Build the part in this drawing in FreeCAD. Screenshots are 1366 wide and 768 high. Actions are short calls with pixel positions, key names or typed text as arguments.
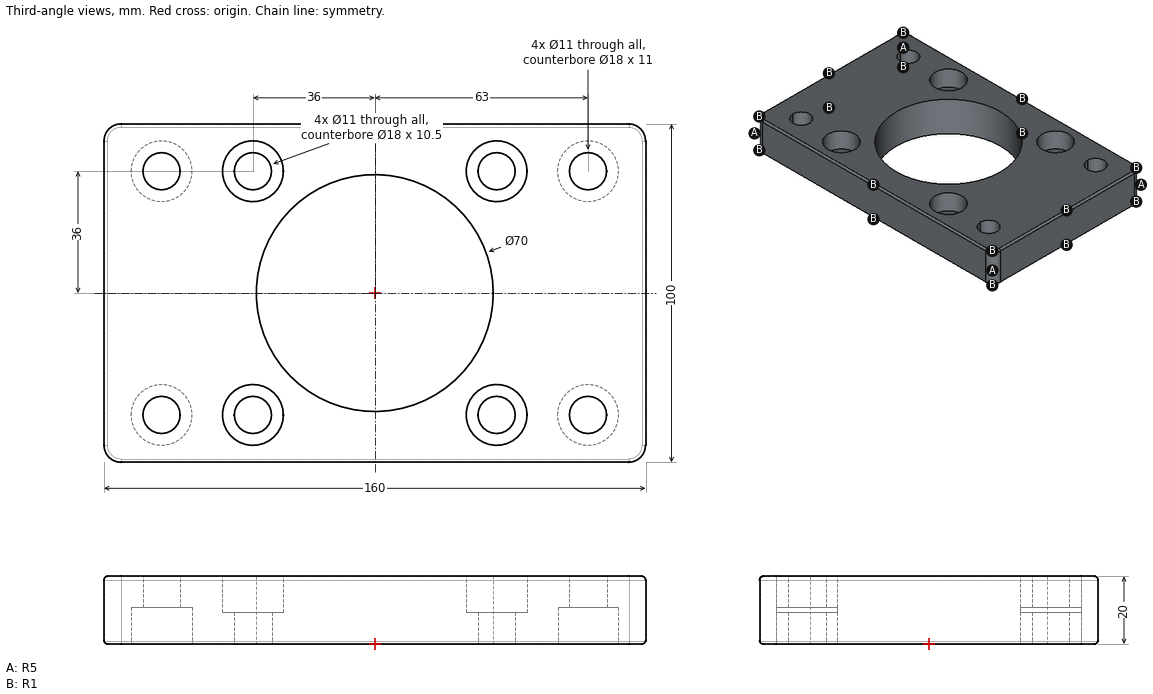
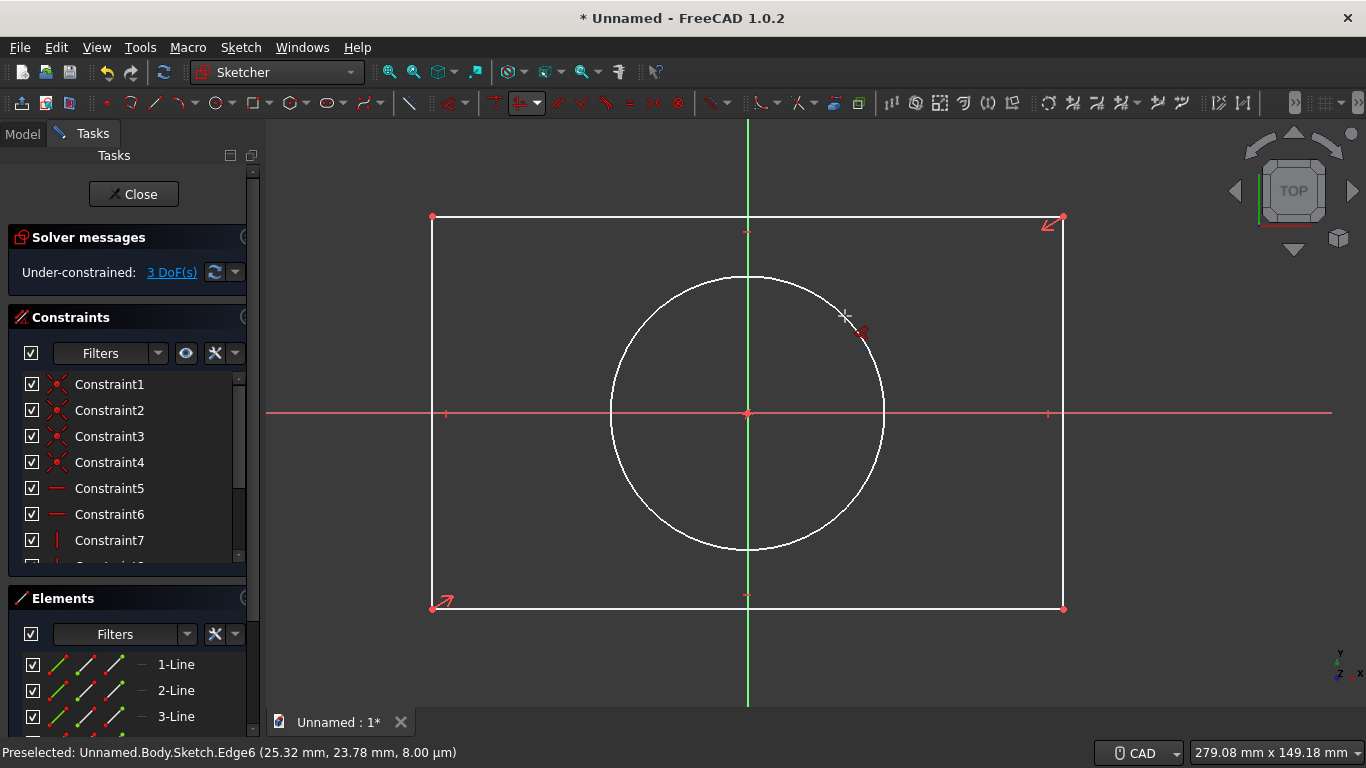
click(844, 316)
click(867, 293)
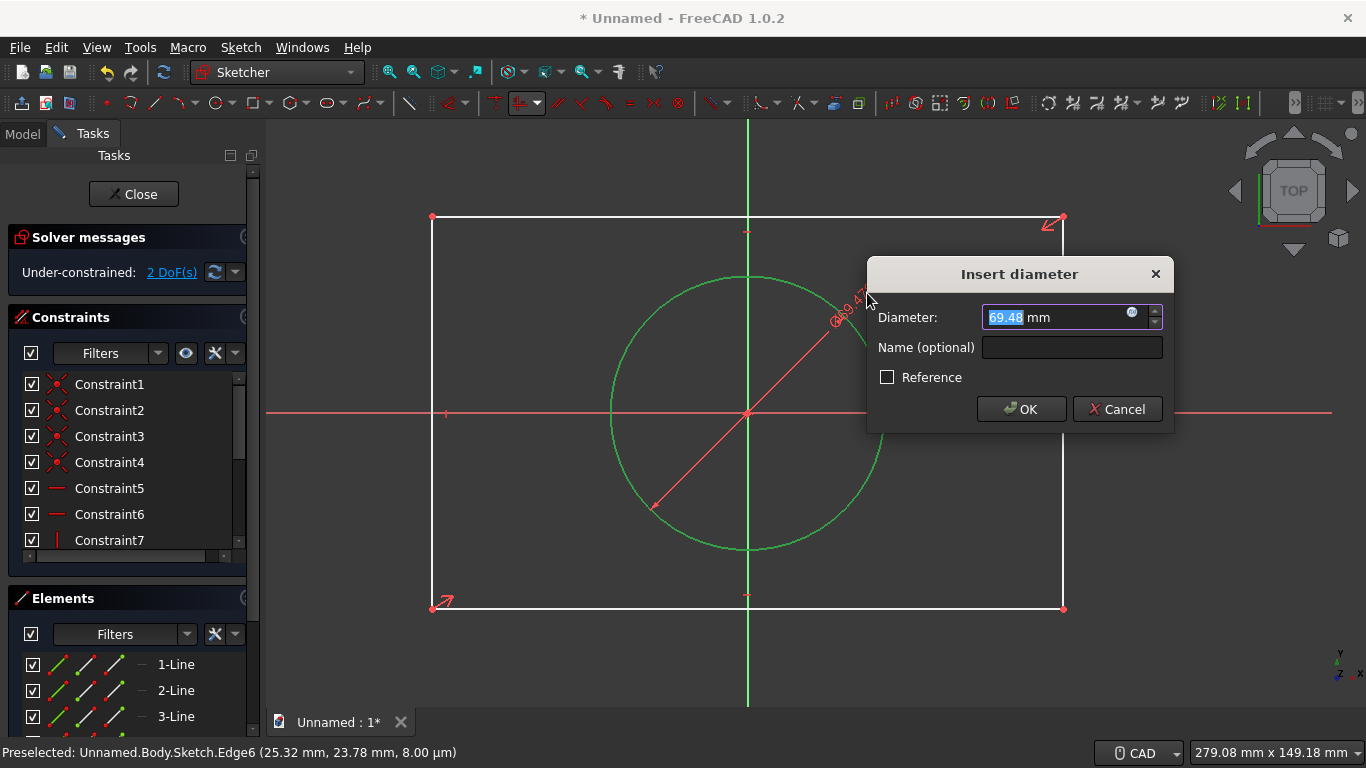
text(70)
key(Return)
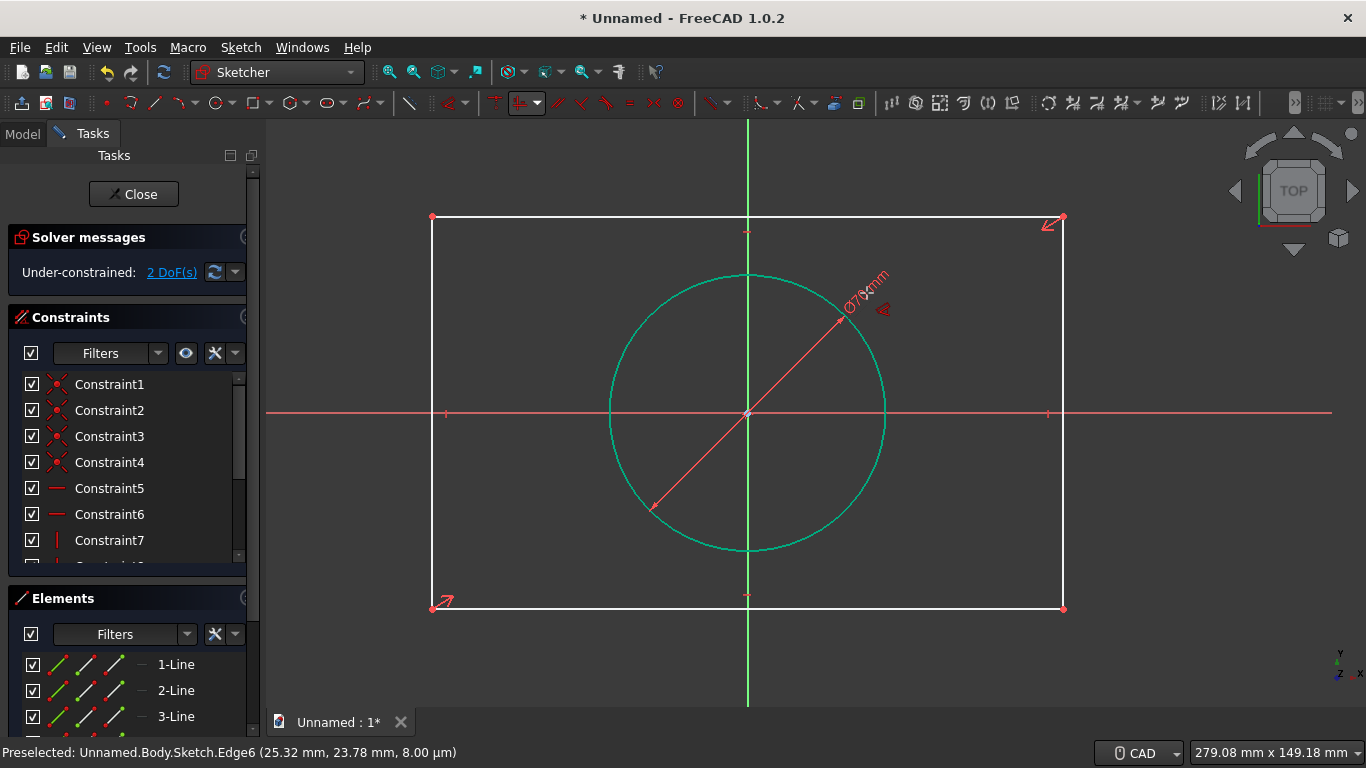
click(621, 609)
click(602, 643)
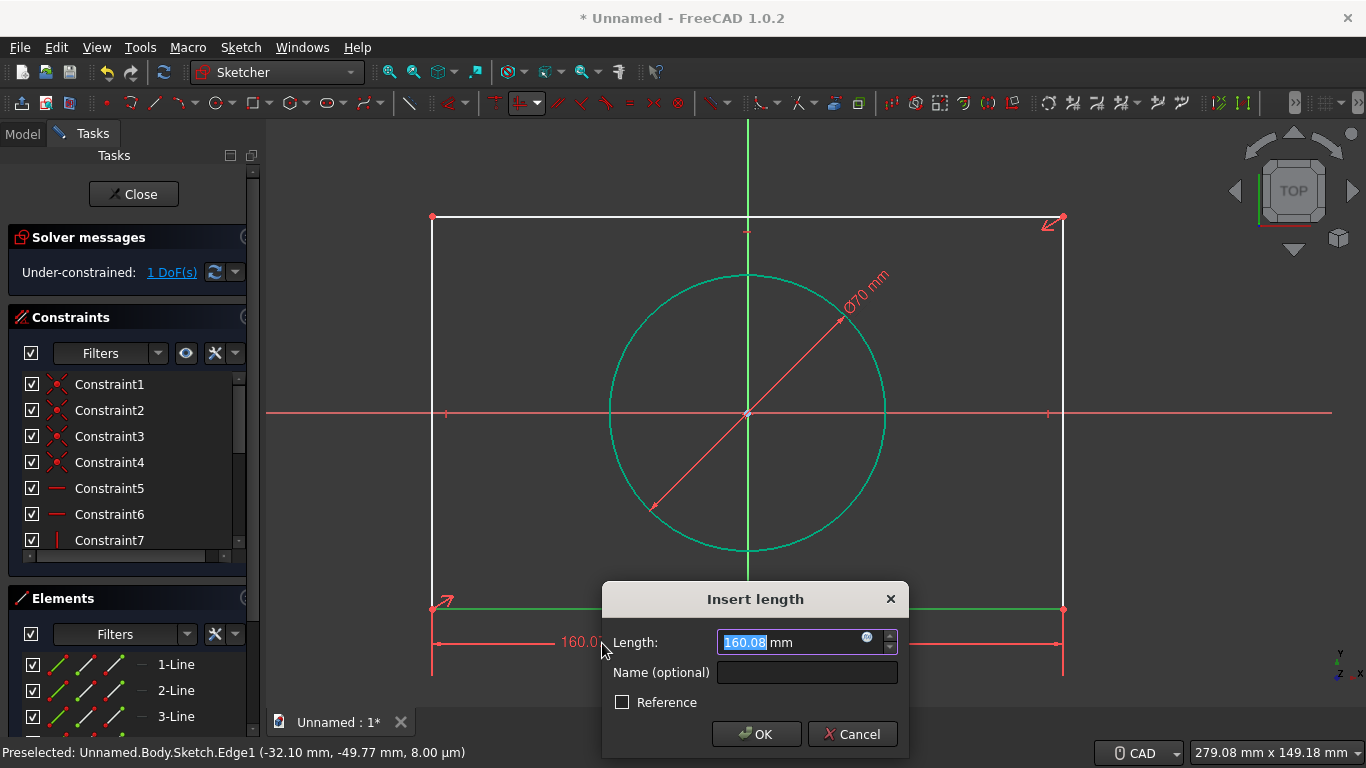
text(160)
key(Return)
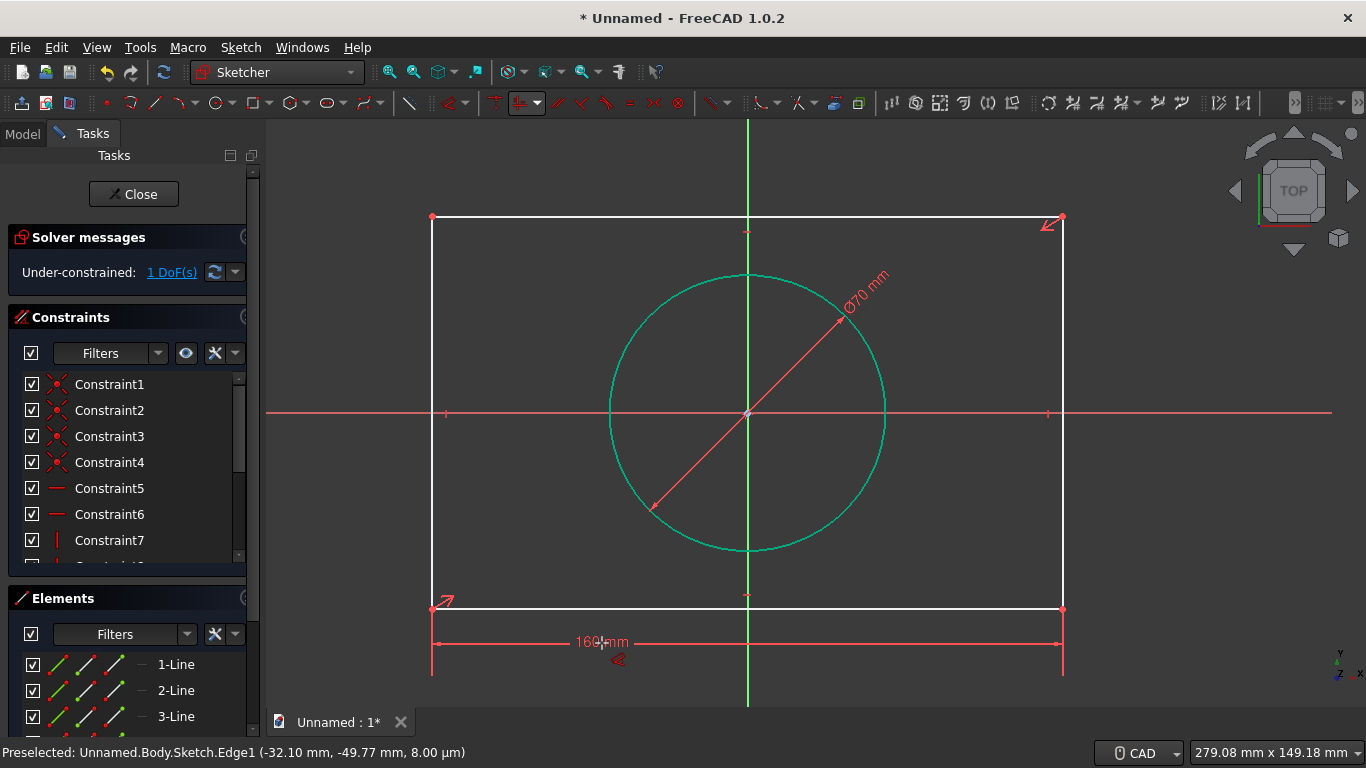
click(1063, 492)
click(1097, 323)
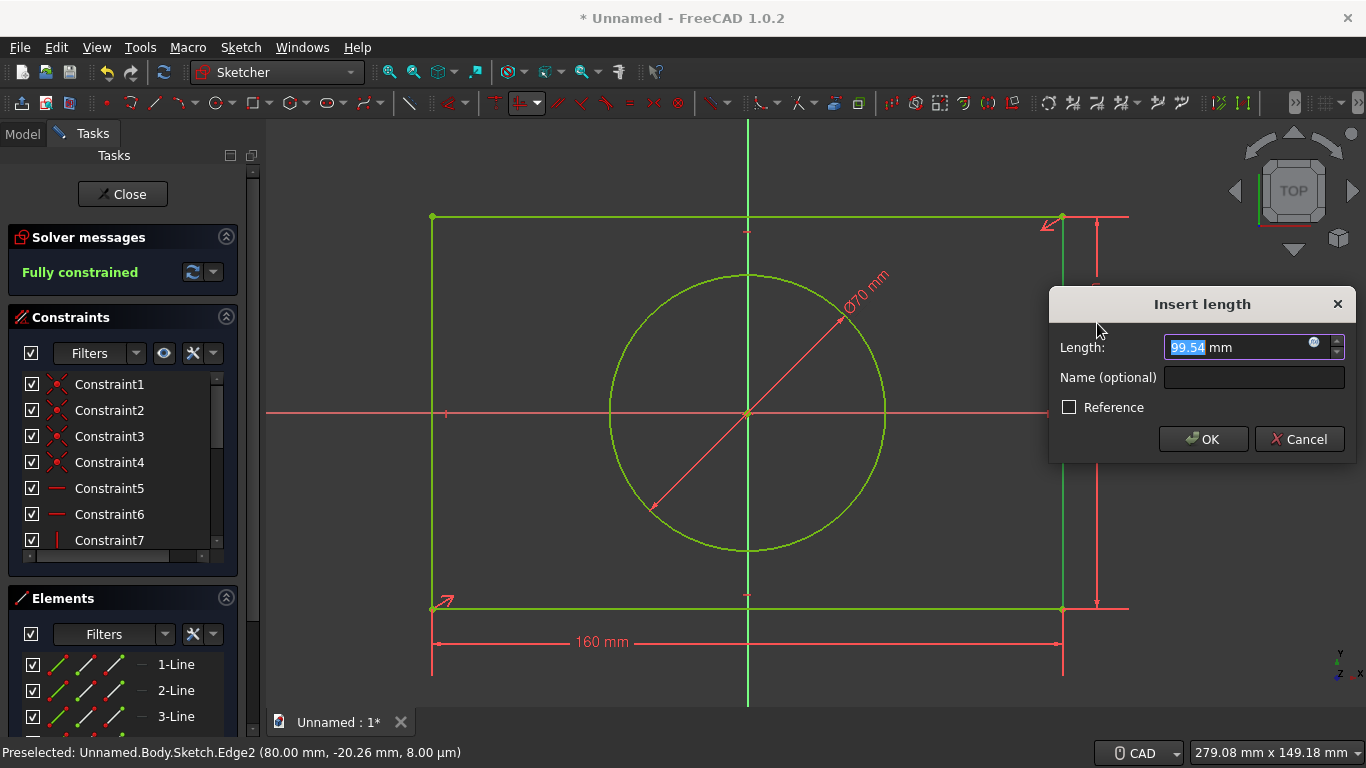
text(100)
key(Return)
key(Escape)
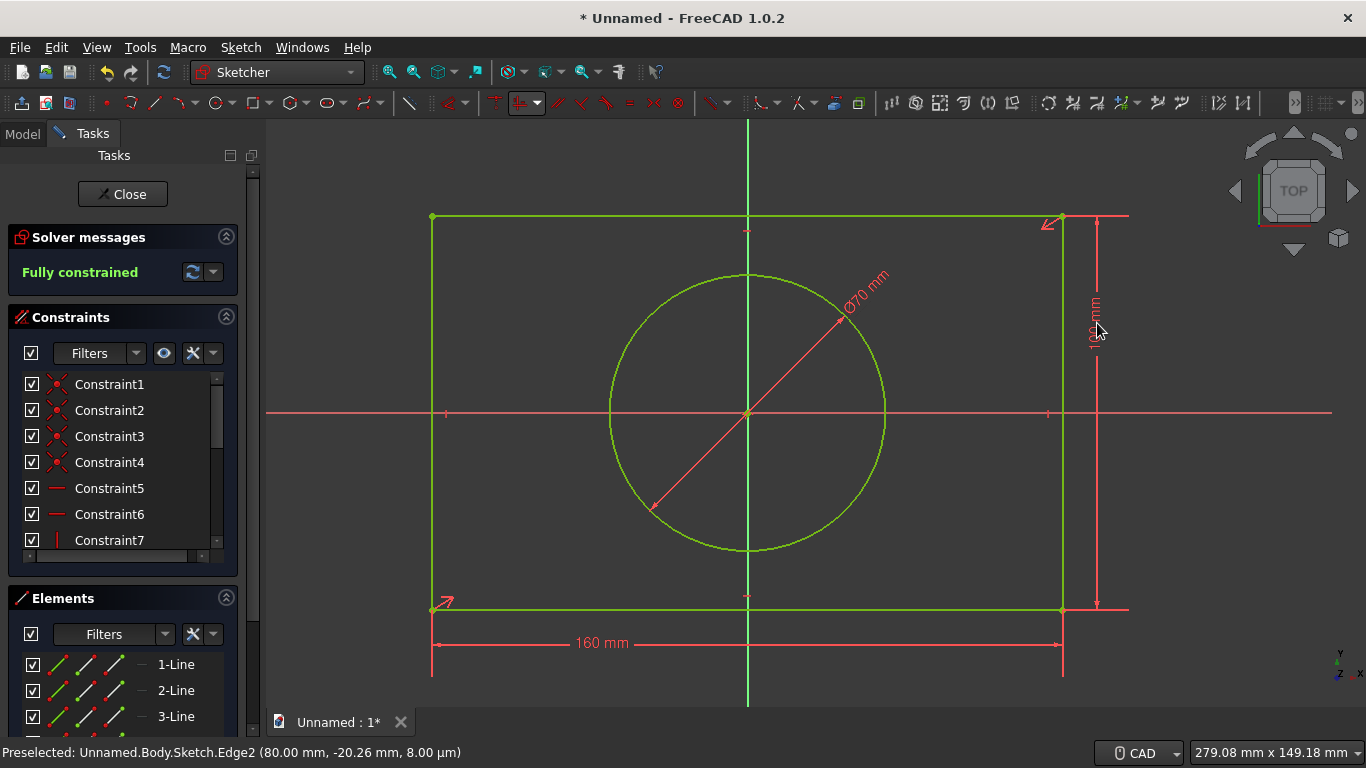
click(123, 194)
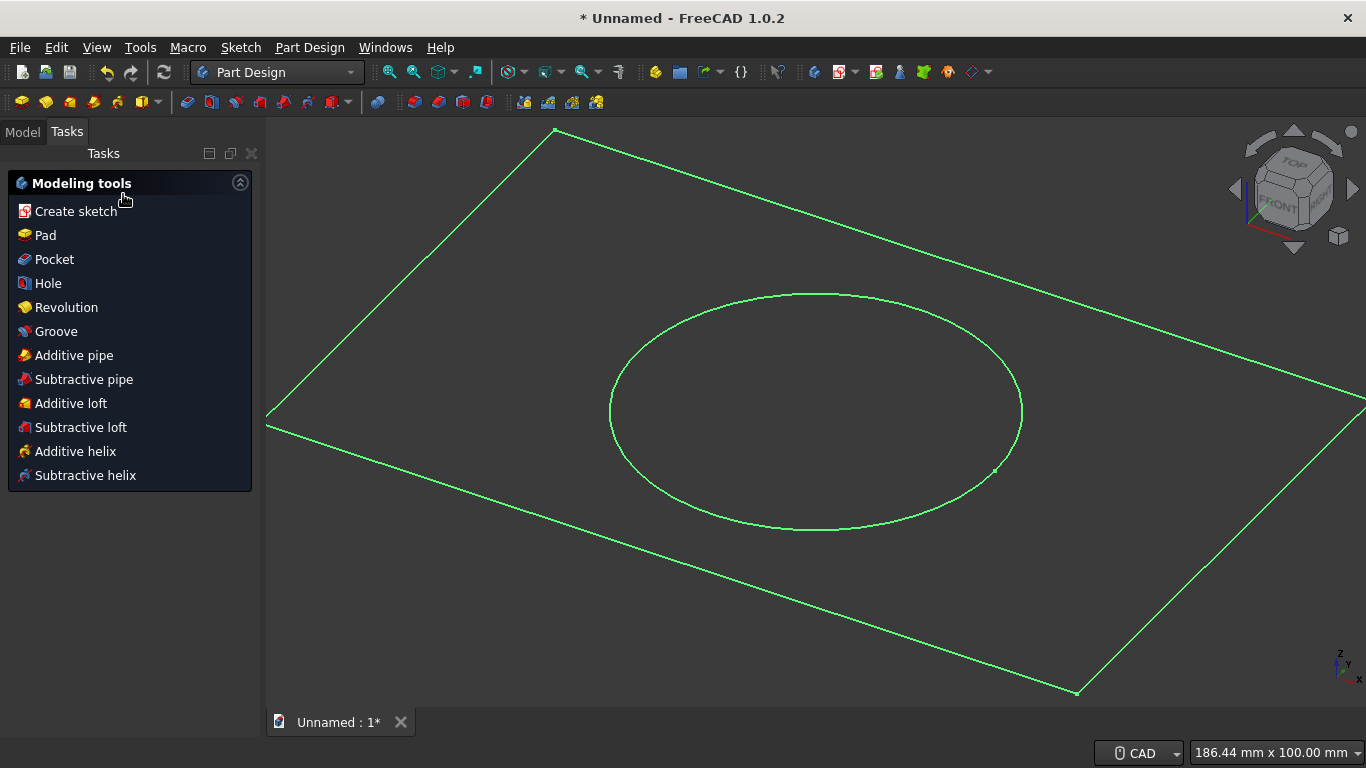
click(22, 102)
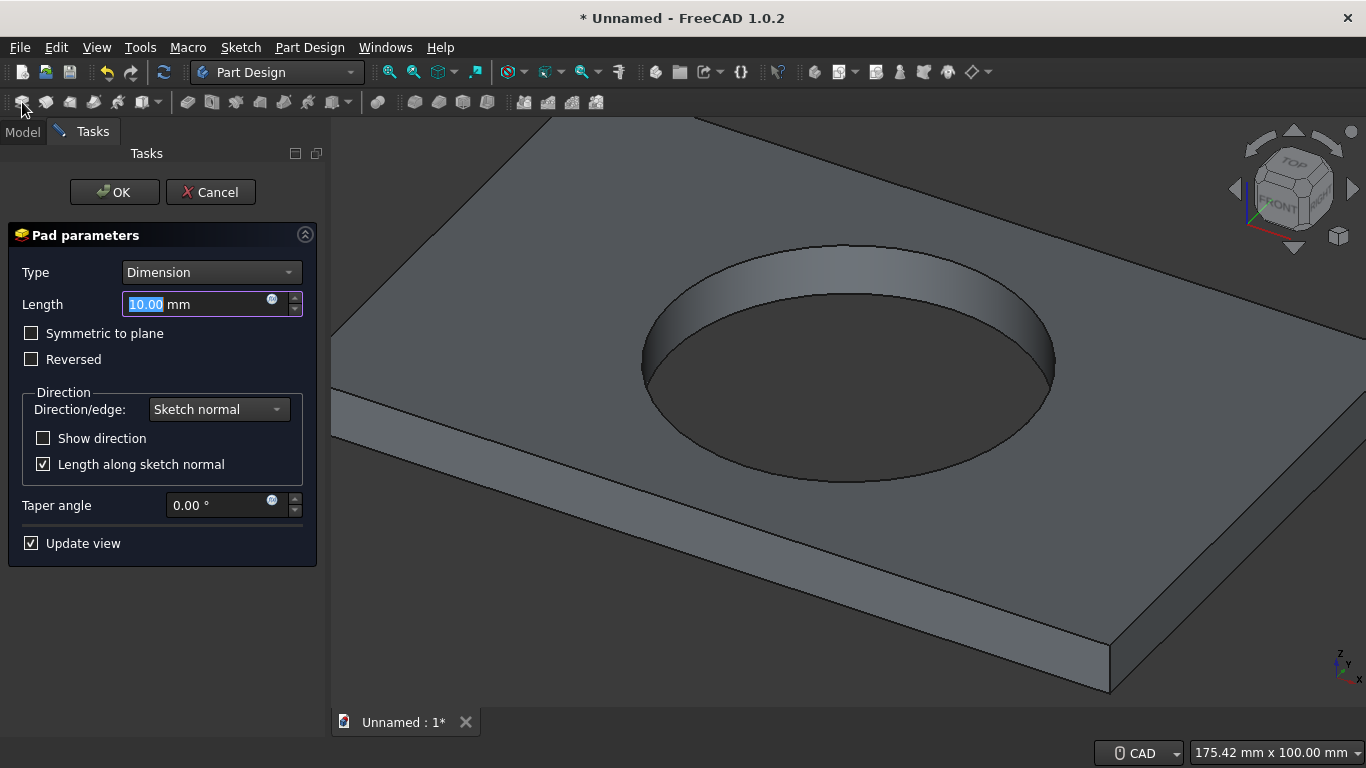
text(20)
key(Tab)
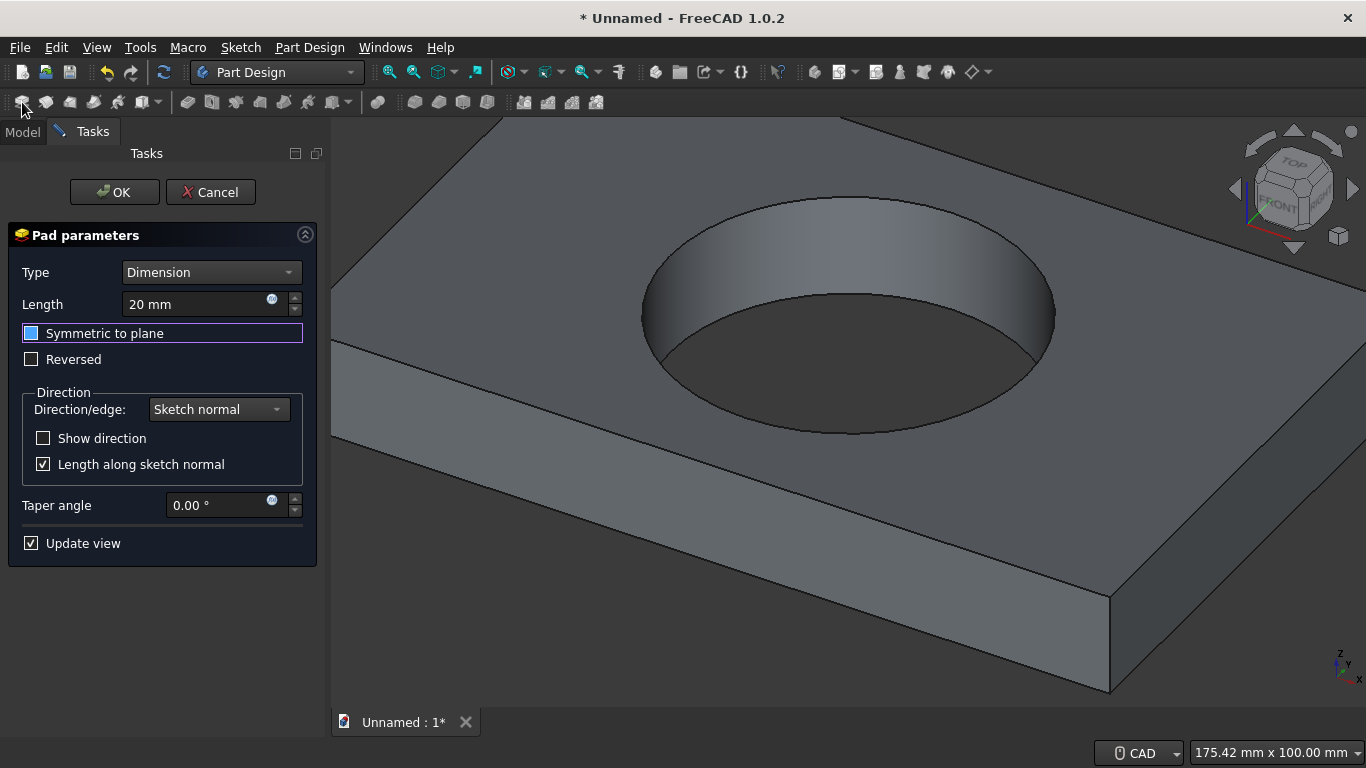
click(115, 192)